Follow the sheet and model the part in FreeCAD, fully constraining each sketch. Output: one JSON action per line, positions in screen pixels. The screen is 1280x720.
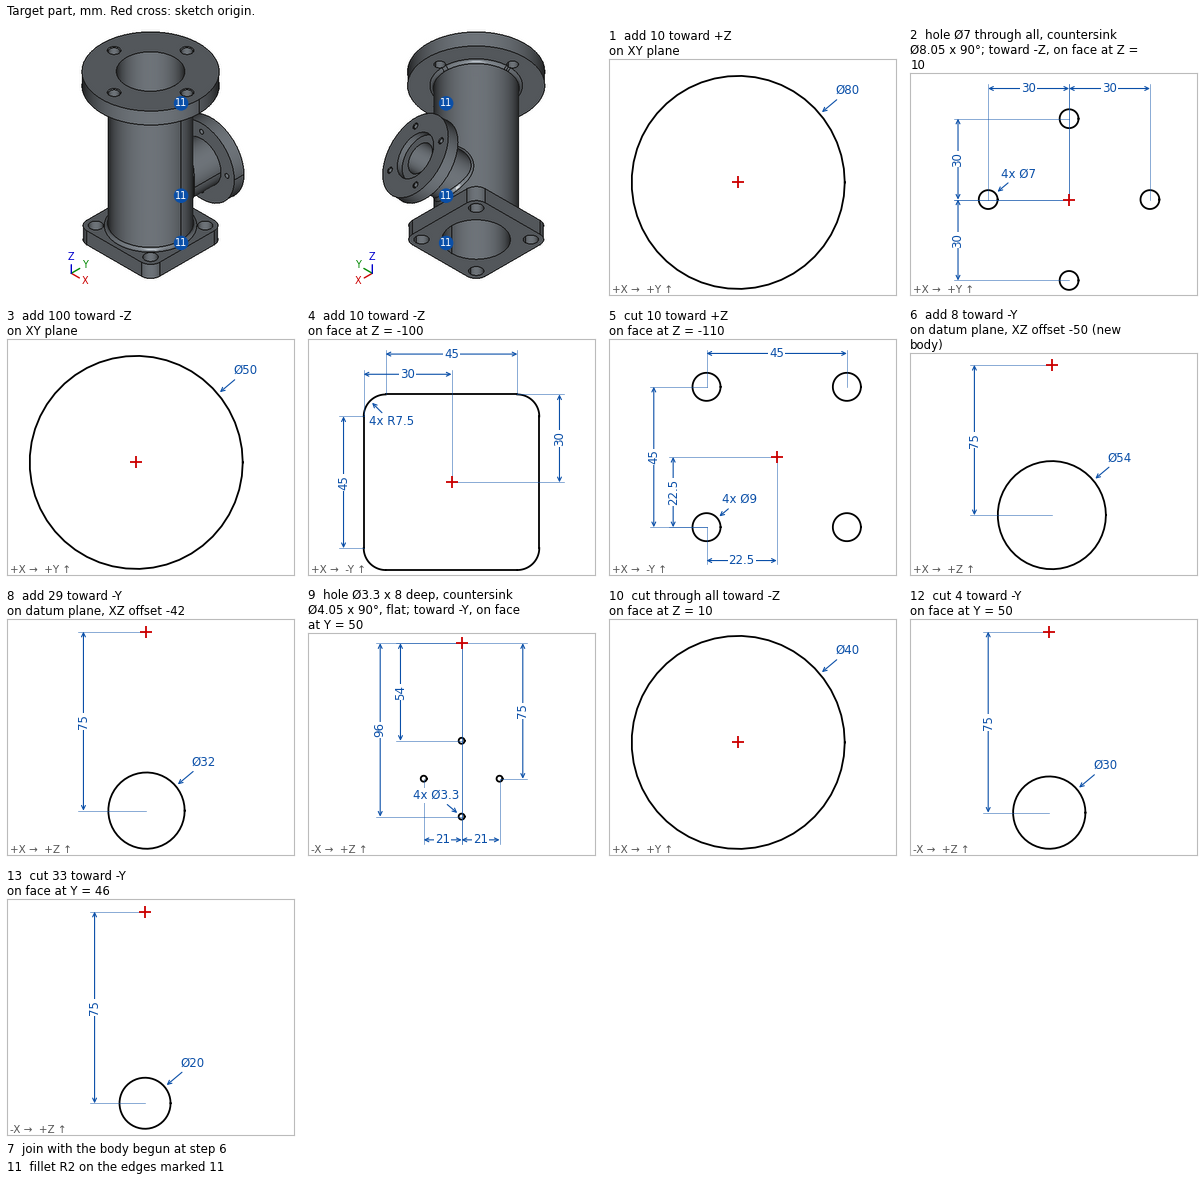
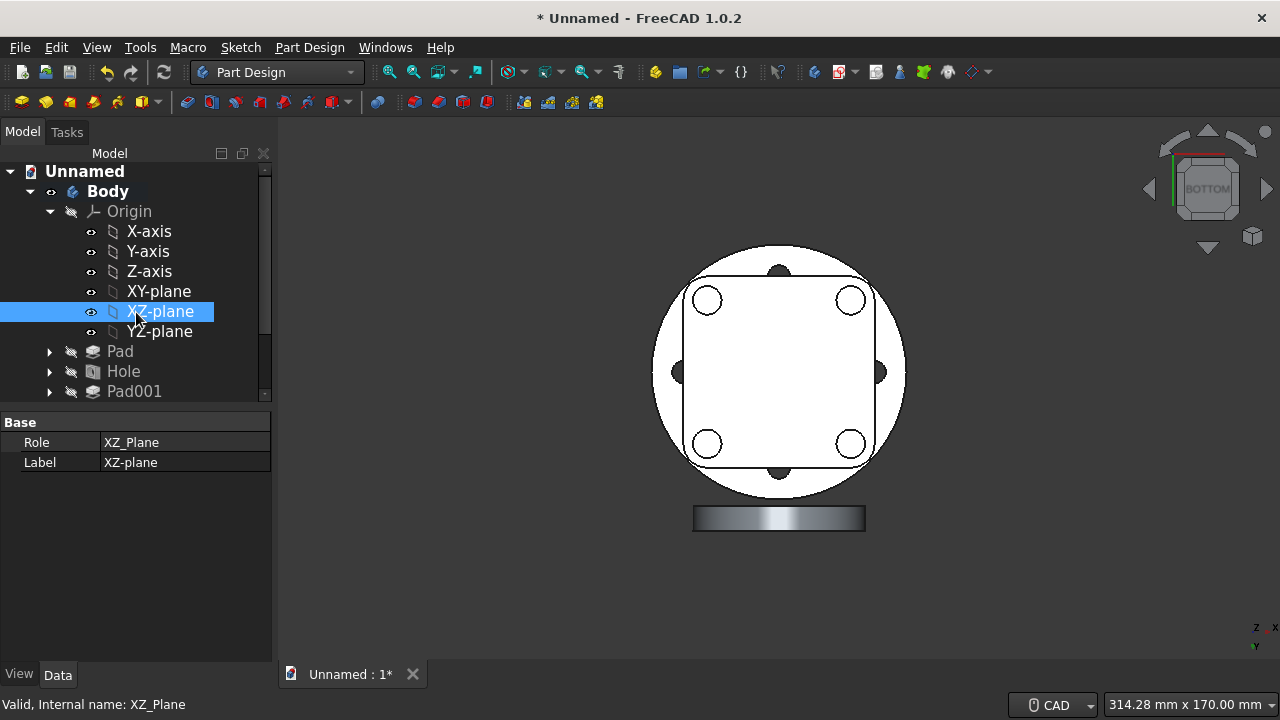
{"action": "left_click", "coordinate": [972, 72]}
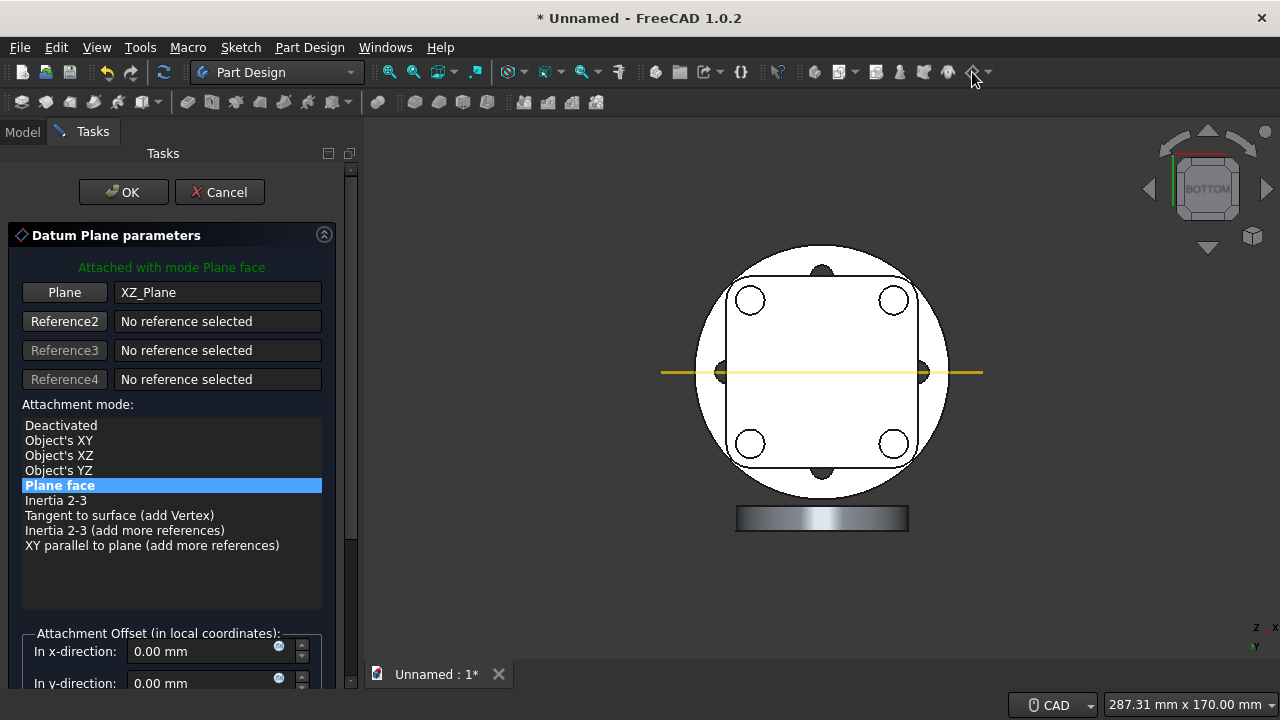
{"action": "scroll", "coordinate": [351, 426], "scroll_direction": "down", "scroll_amount": 2}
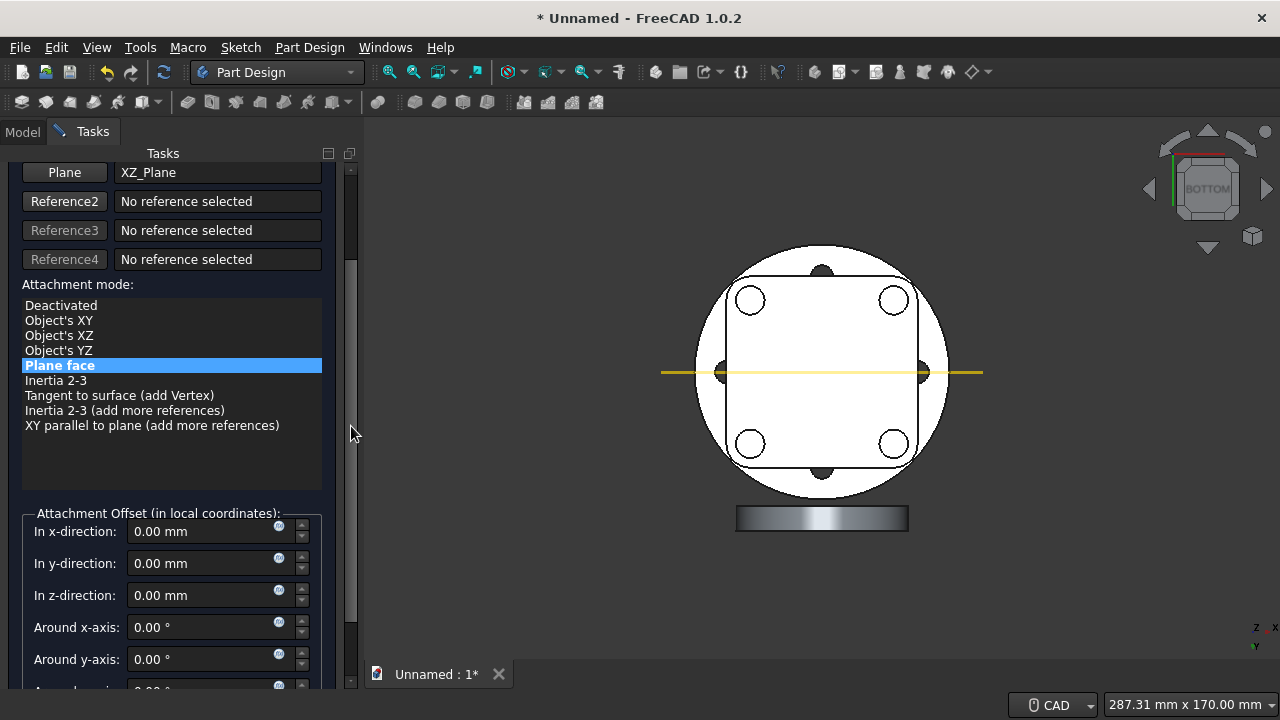
{"action": "triple_click", "coordinate": [210, 595]}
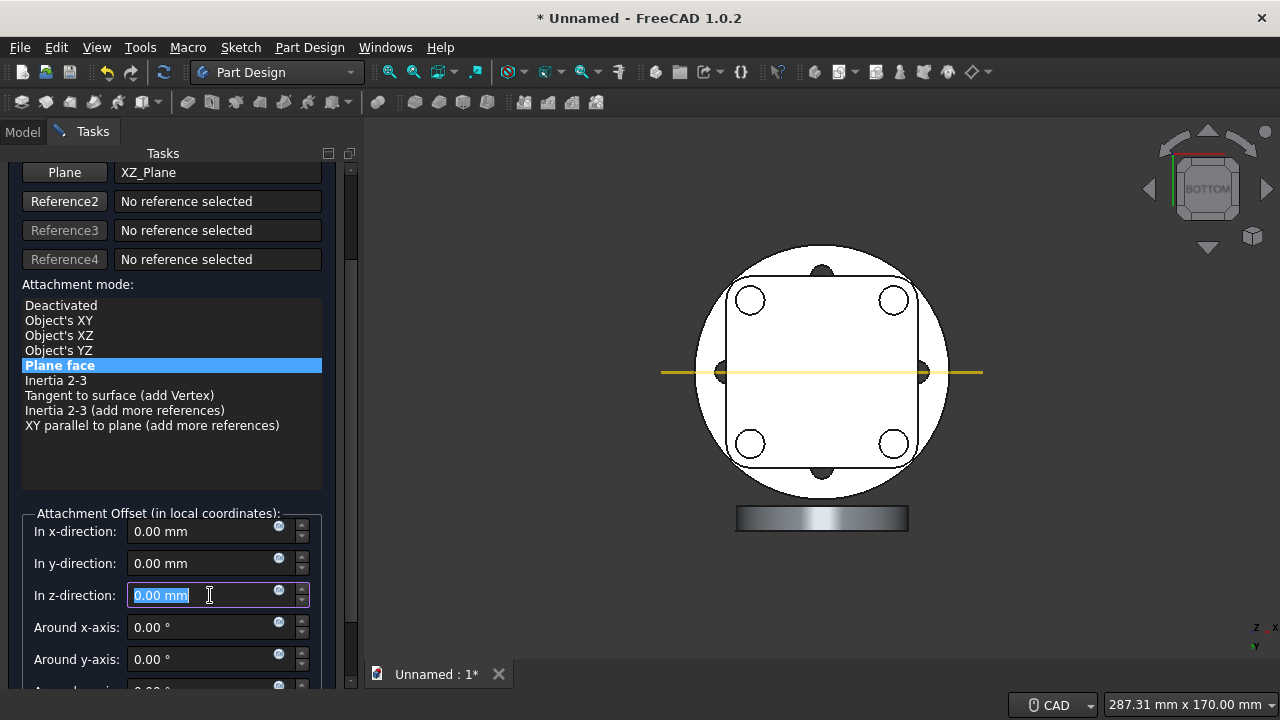
{"action": "type", "text": "-42"}
{"action": "key", "text": "Tab"}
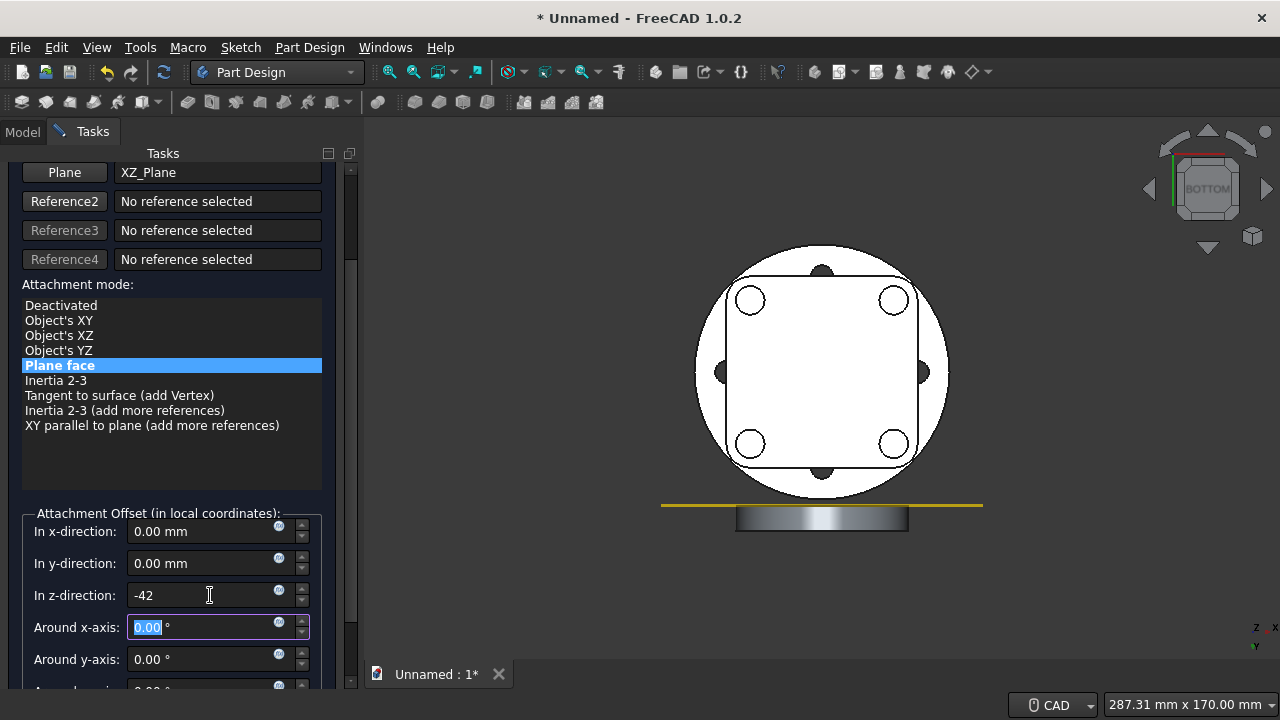
{"action": "scroll", "coordinate": [351, 426], "scroll_direction": "up", "scroll_amount": 3}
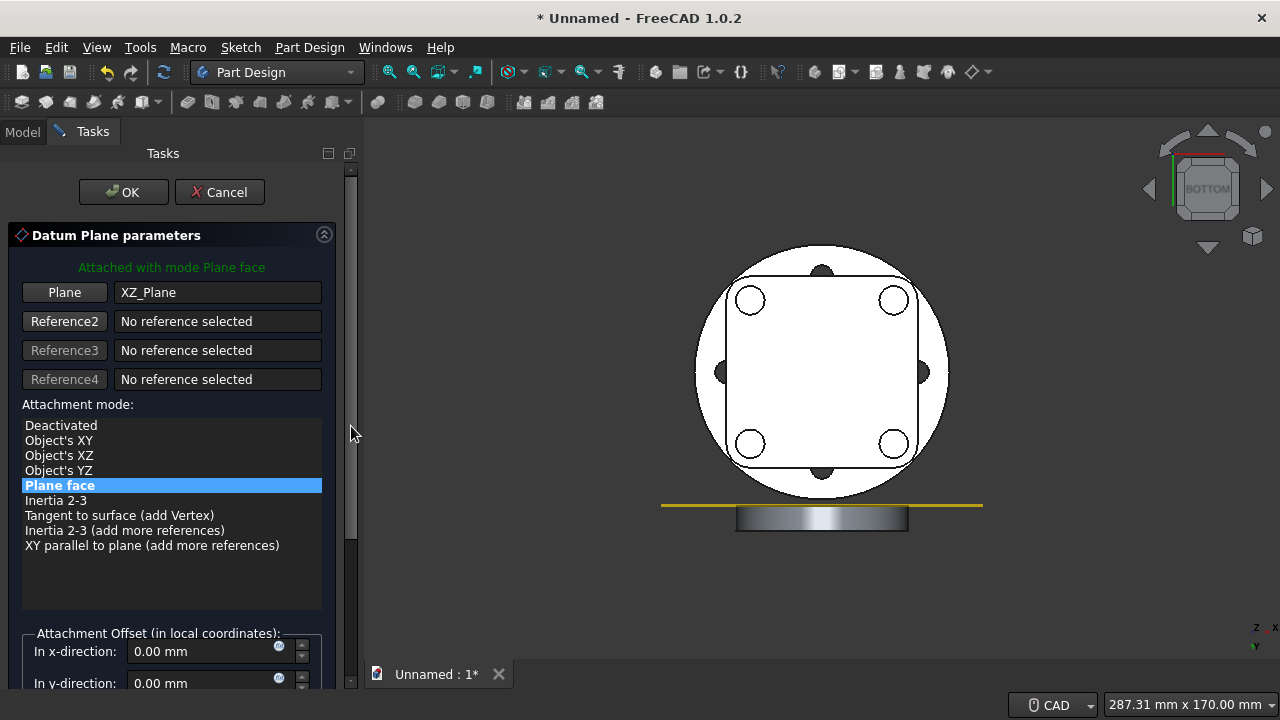
{"action": "left_click", "coordinate": [124, 192]}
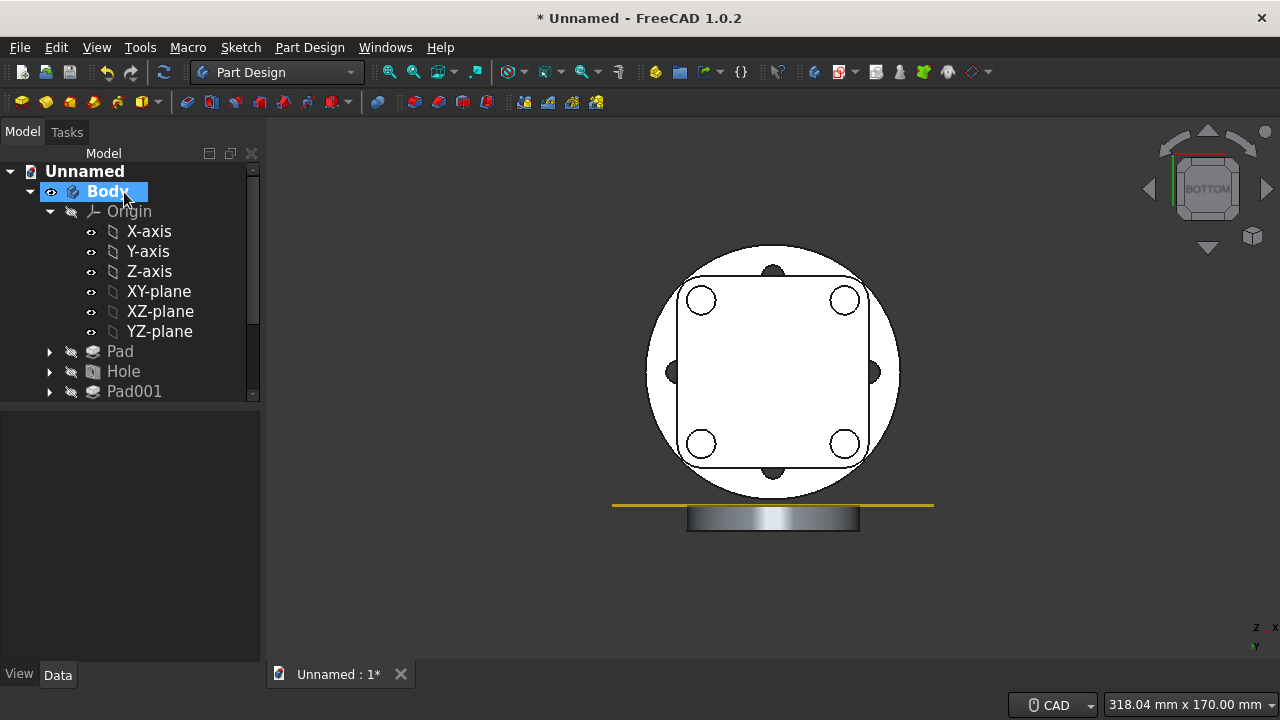
{"action": "scroll", "coordinate": [100, 287], "scroll_direction": "down", "scroll_amount": 3}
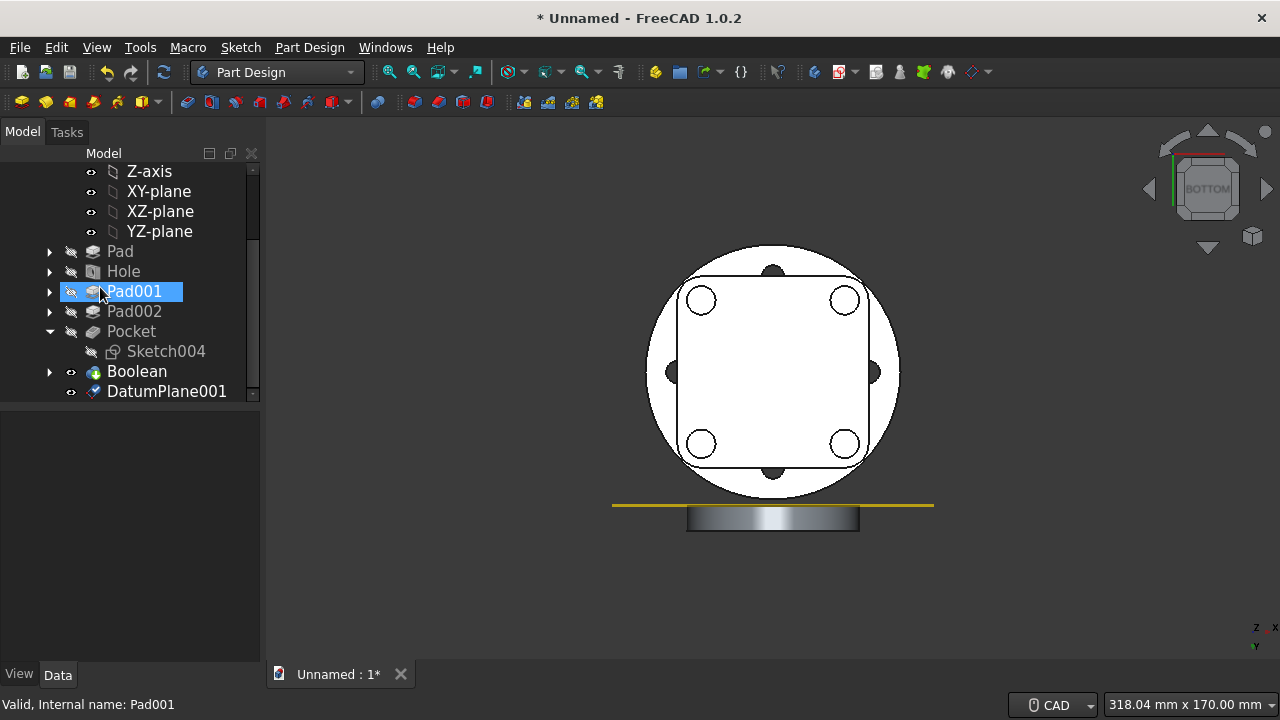
{"action": "left_click", "coordinate": [116, 392]}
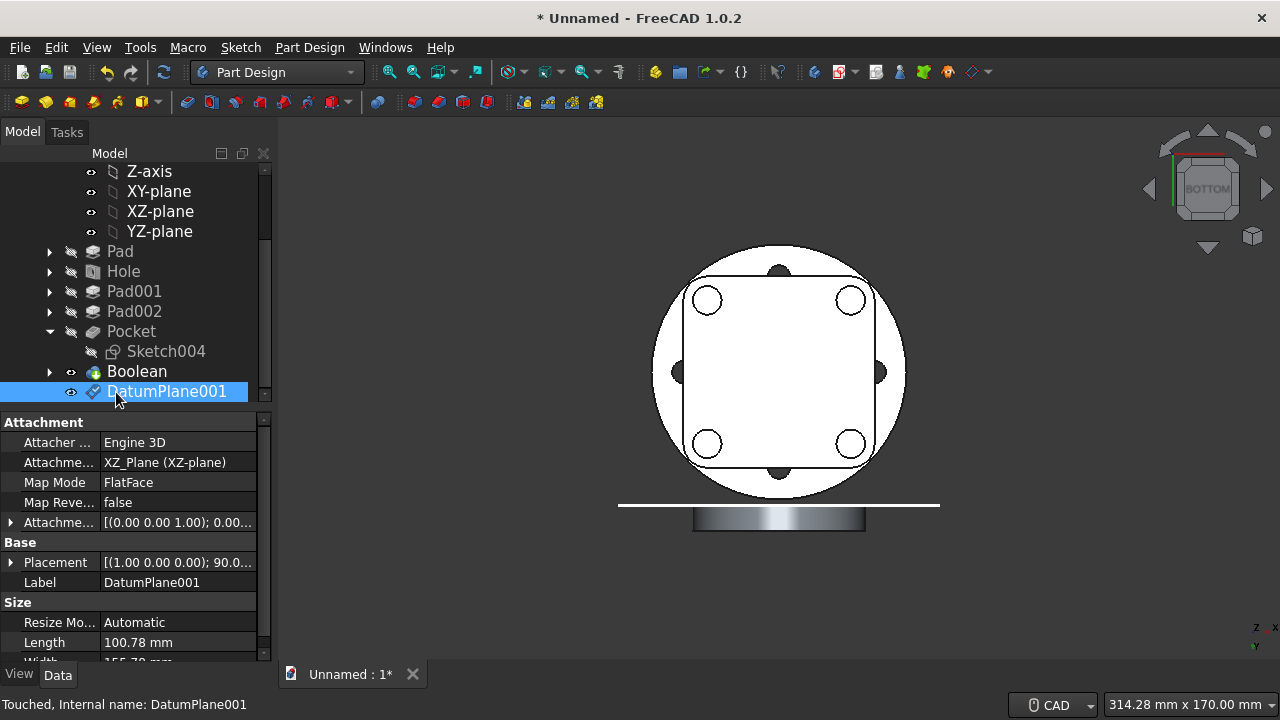
{"action": "left_click", "coordinate": [840, 72]}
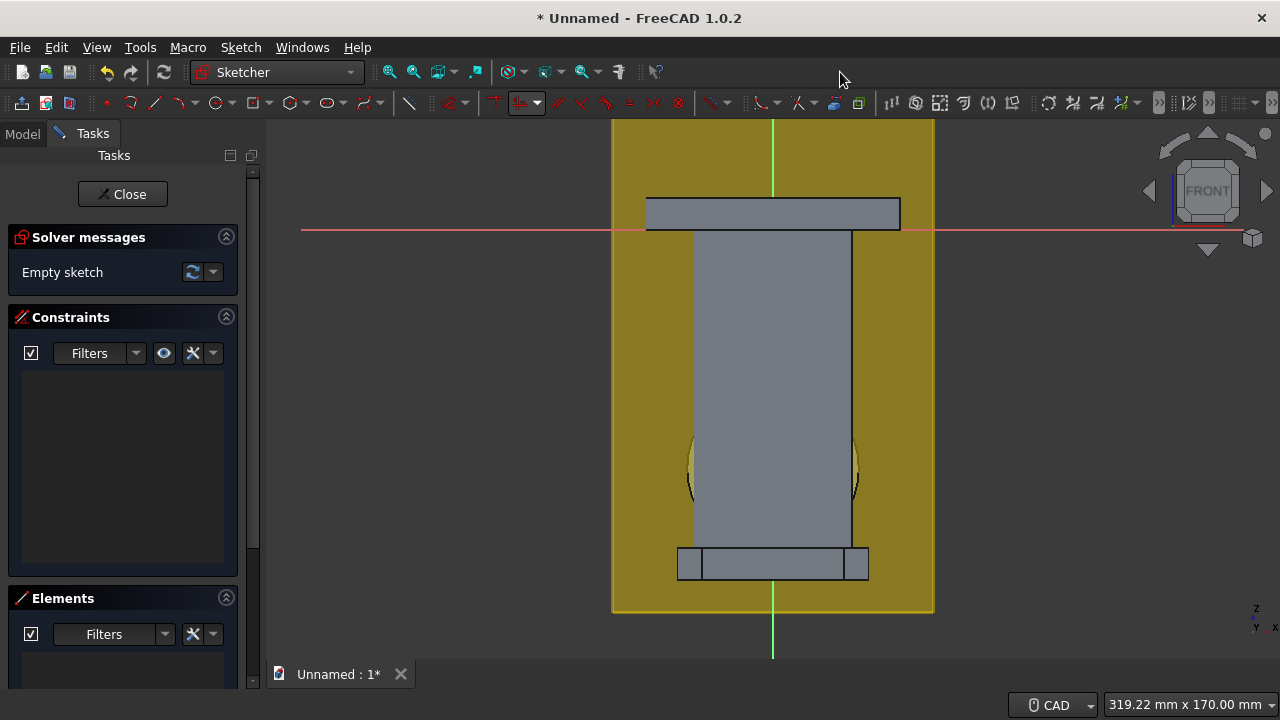
{"action": "left_click", "coordinate": [70, 104]}